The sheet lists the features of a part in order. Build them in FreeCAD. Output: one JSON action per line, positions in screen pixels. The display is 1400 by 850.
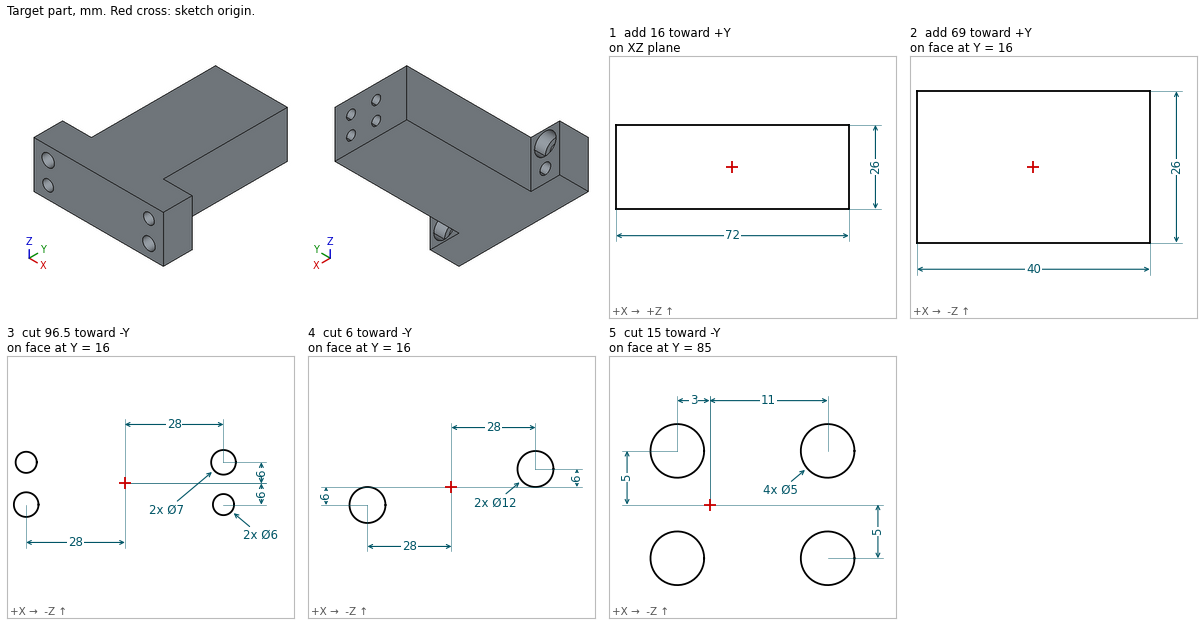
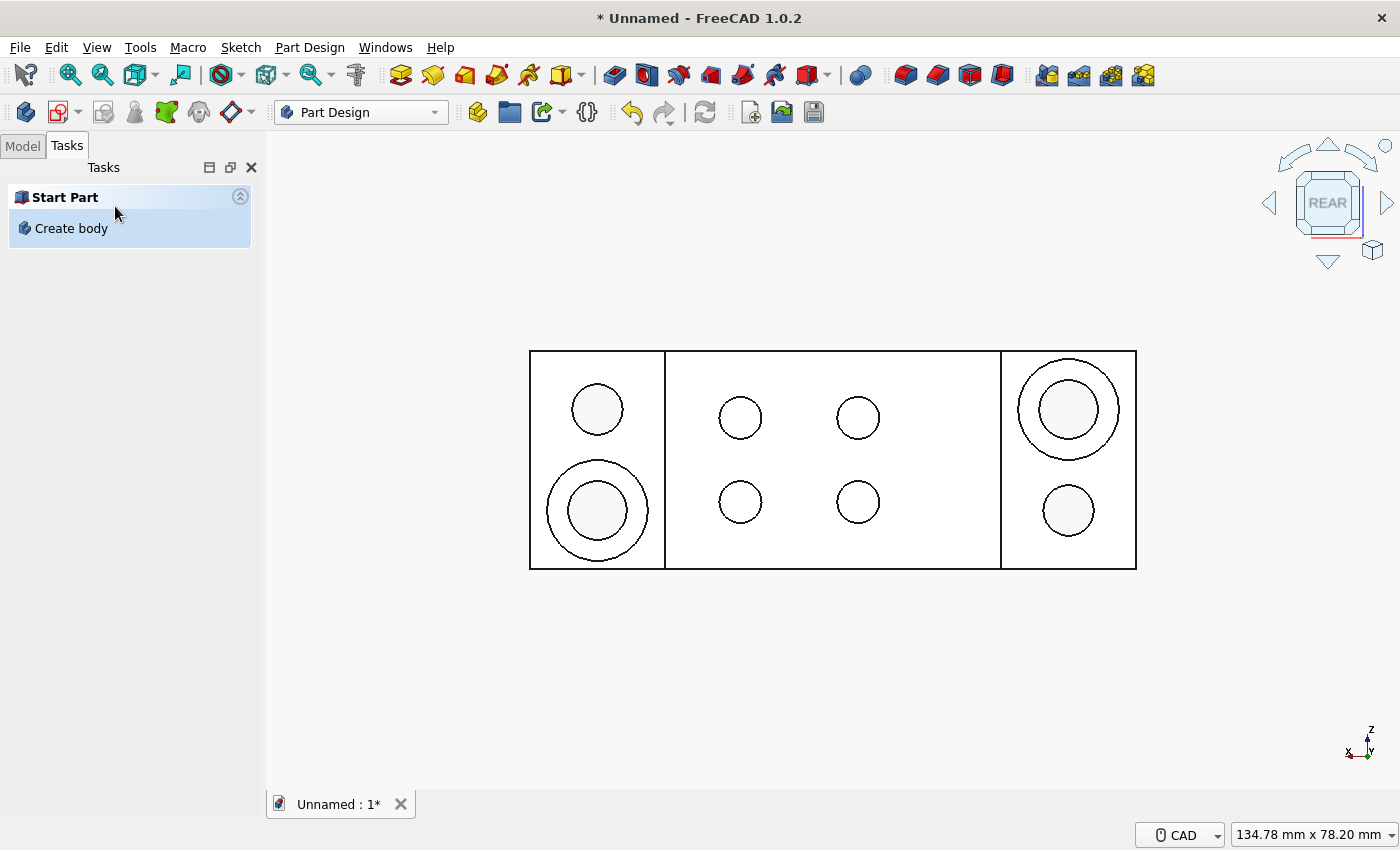
{"action": "key", "text": "0"}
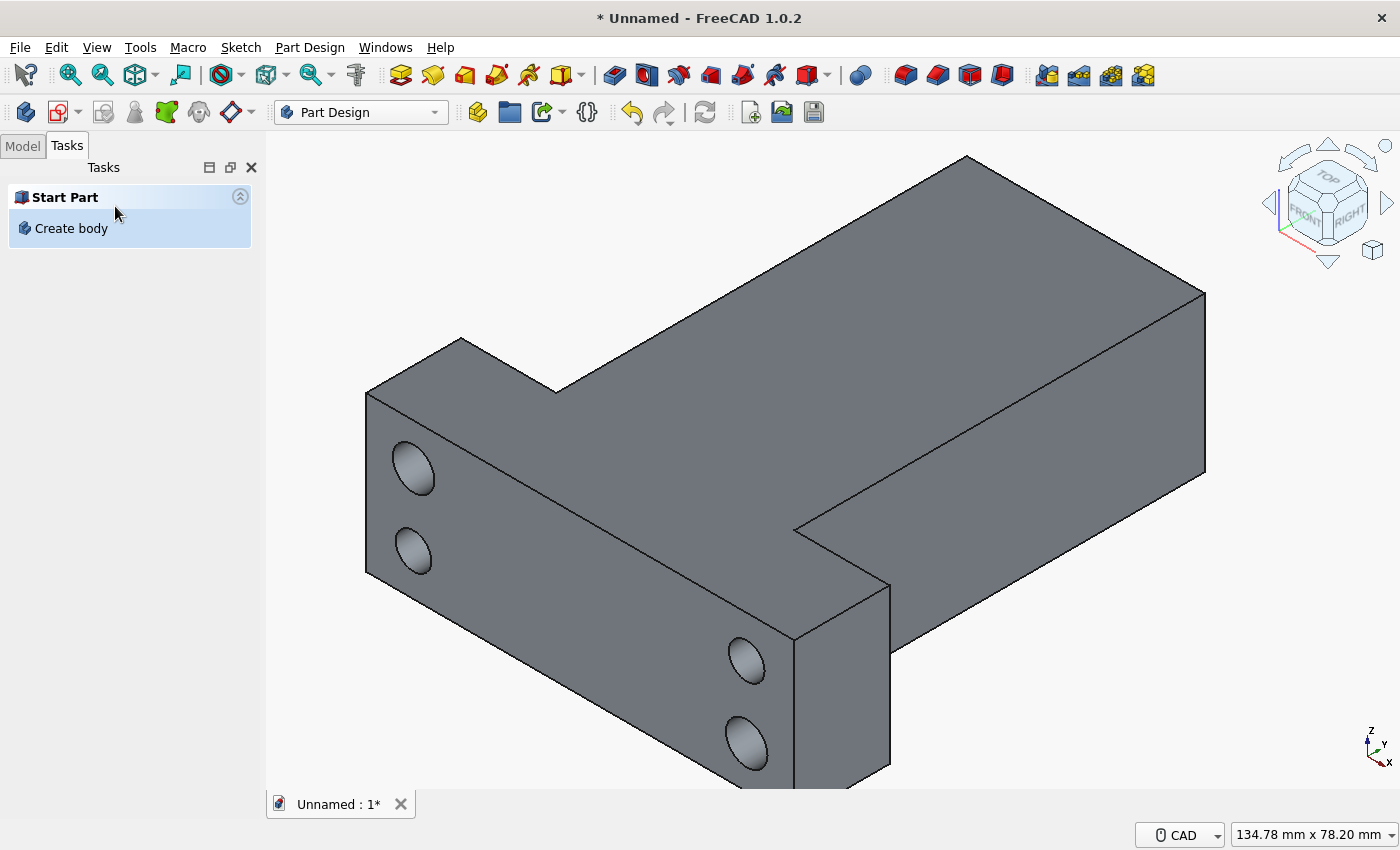
{"action": "key", "text": "v f"}